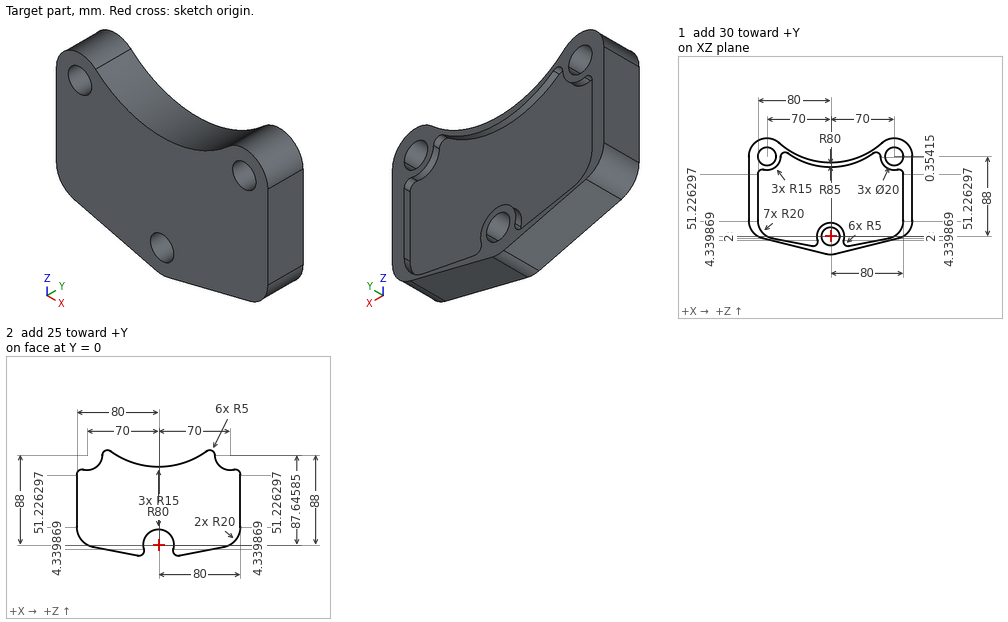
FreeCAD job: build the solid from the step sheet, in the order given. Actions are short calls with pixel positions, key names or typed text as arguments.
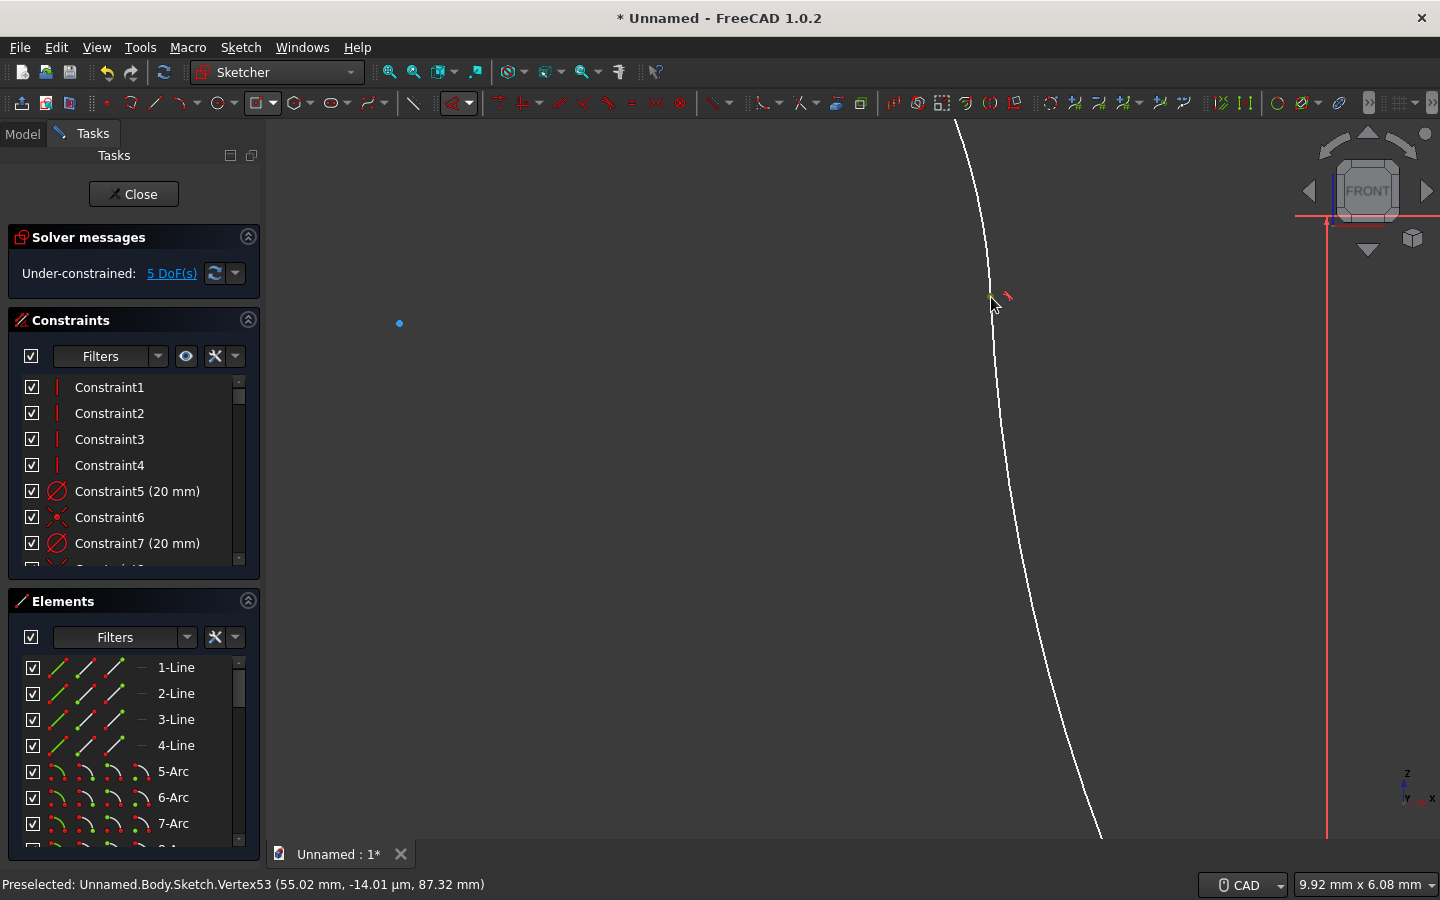
scroll(1053, 264, down, 16)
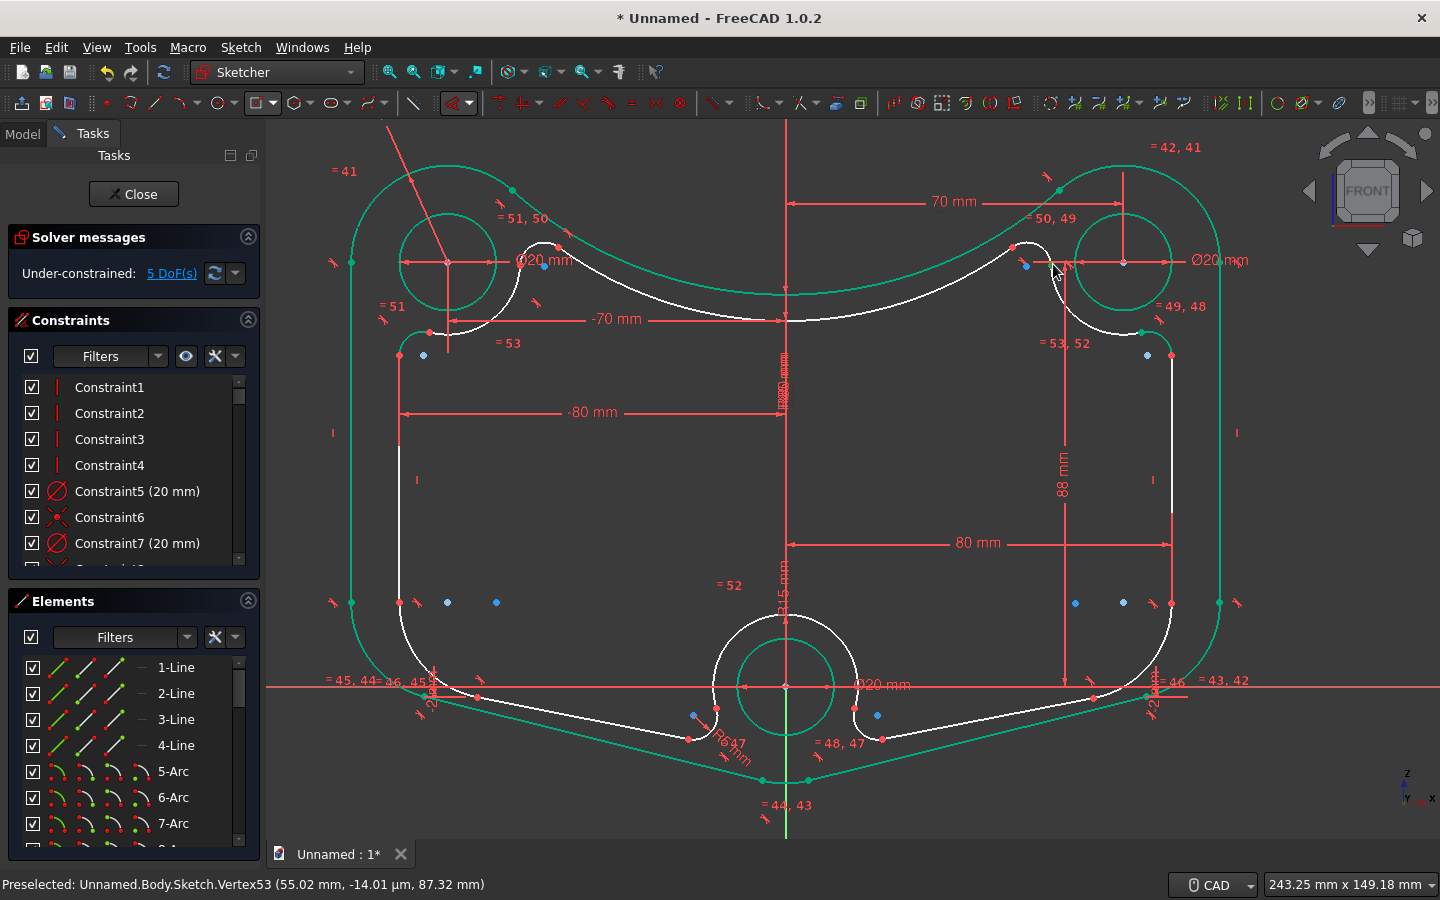
scroll(1123, 262, up, 16)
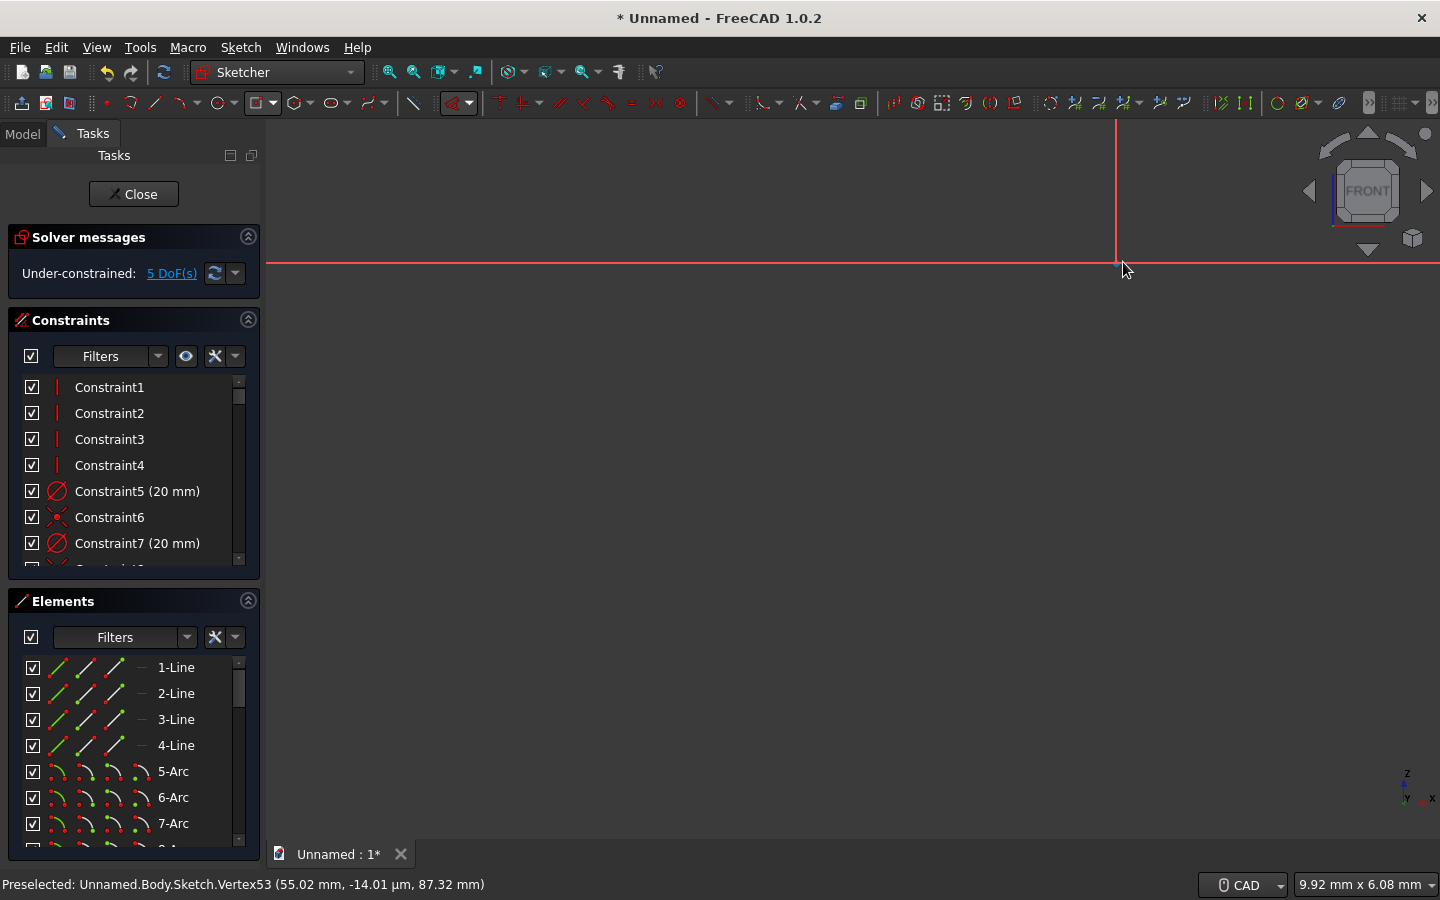
click(1116, 263)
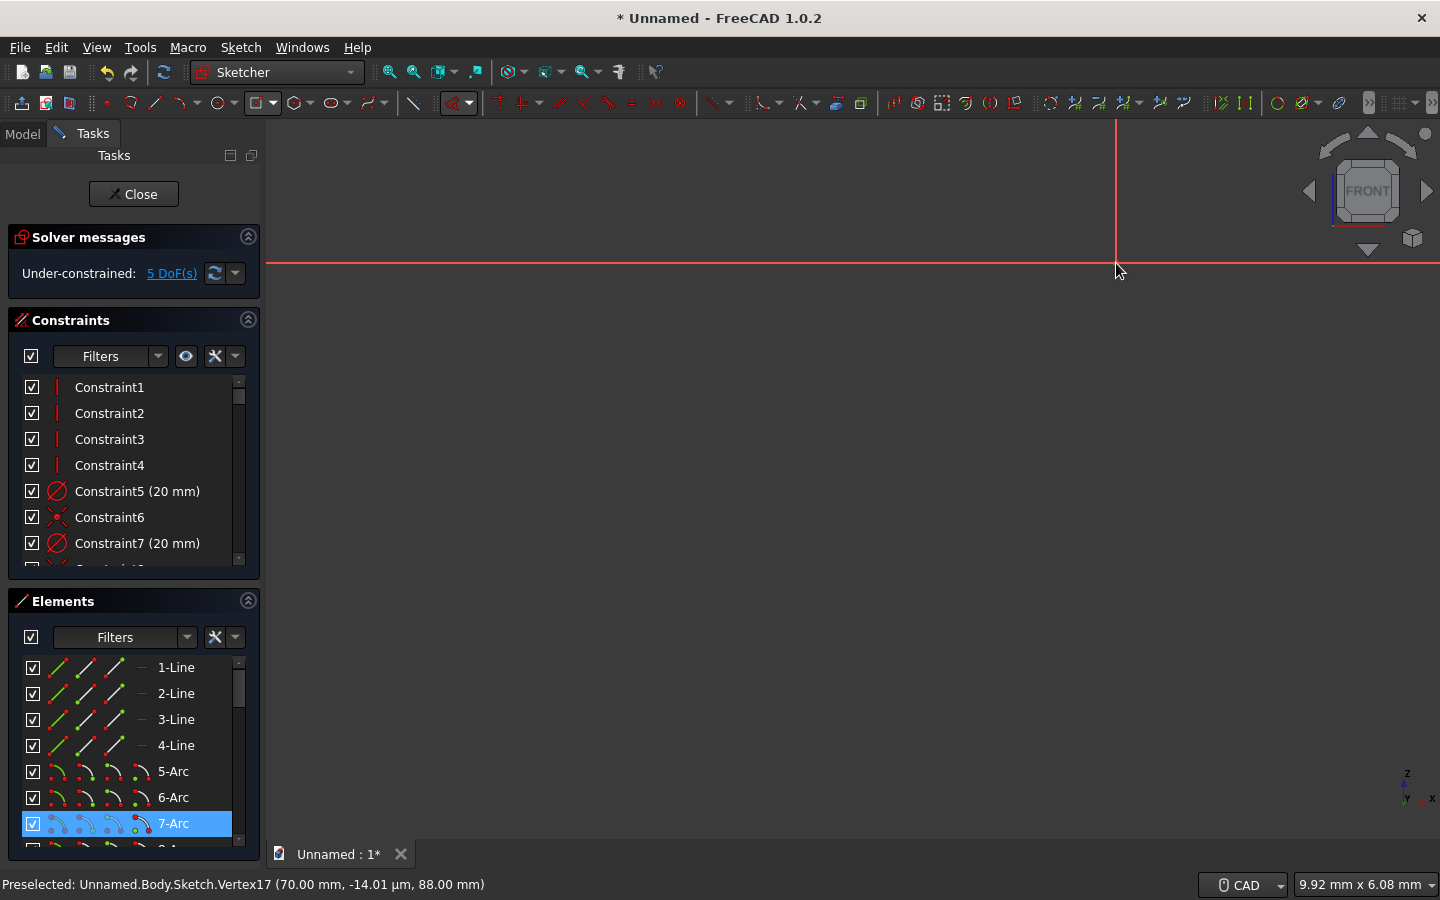
click(472, 104)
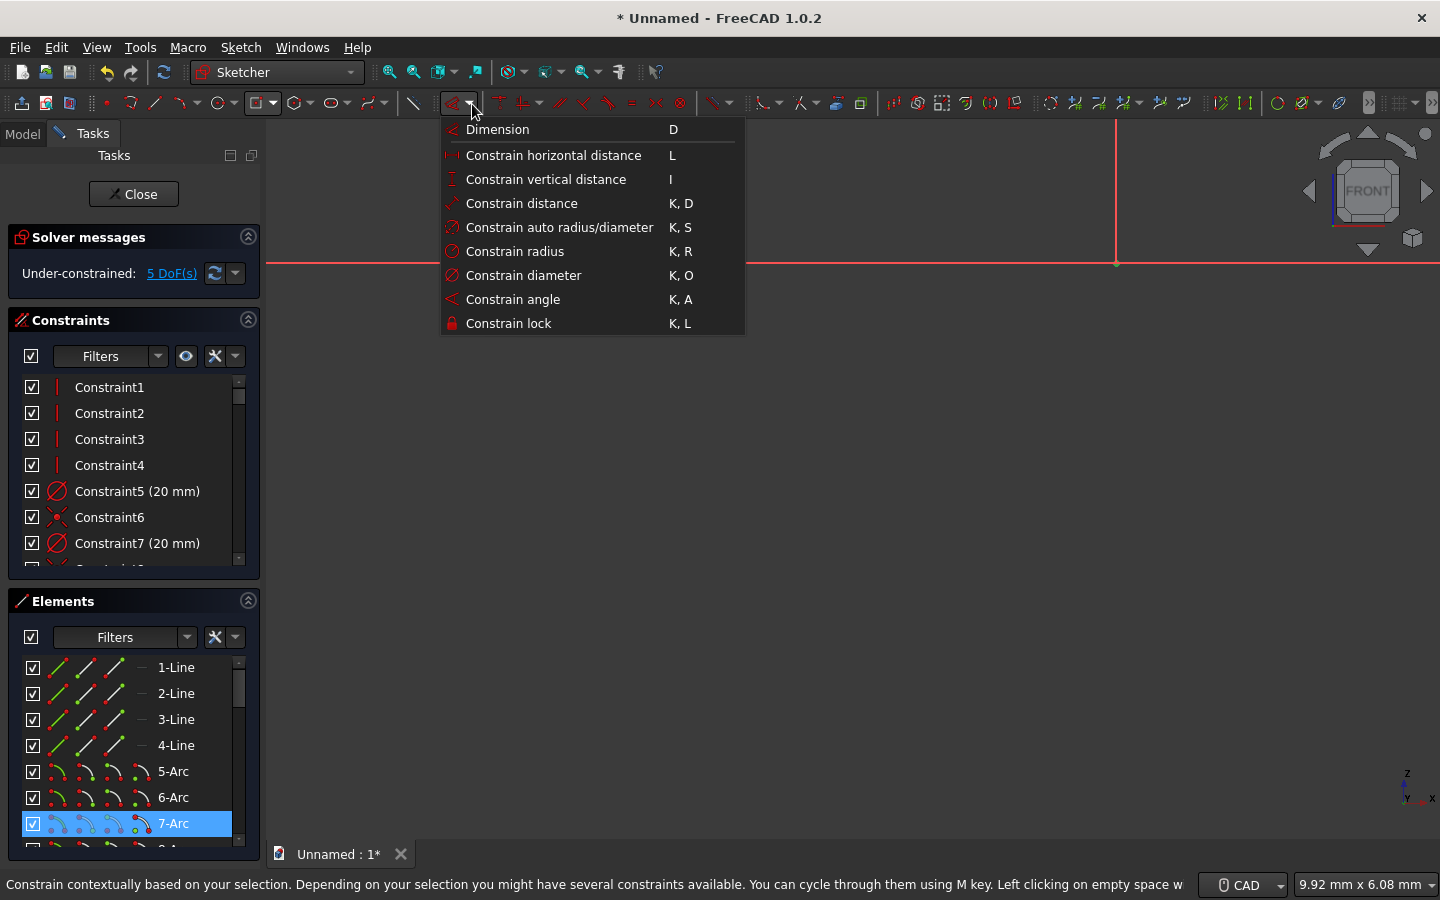
click(593, 179)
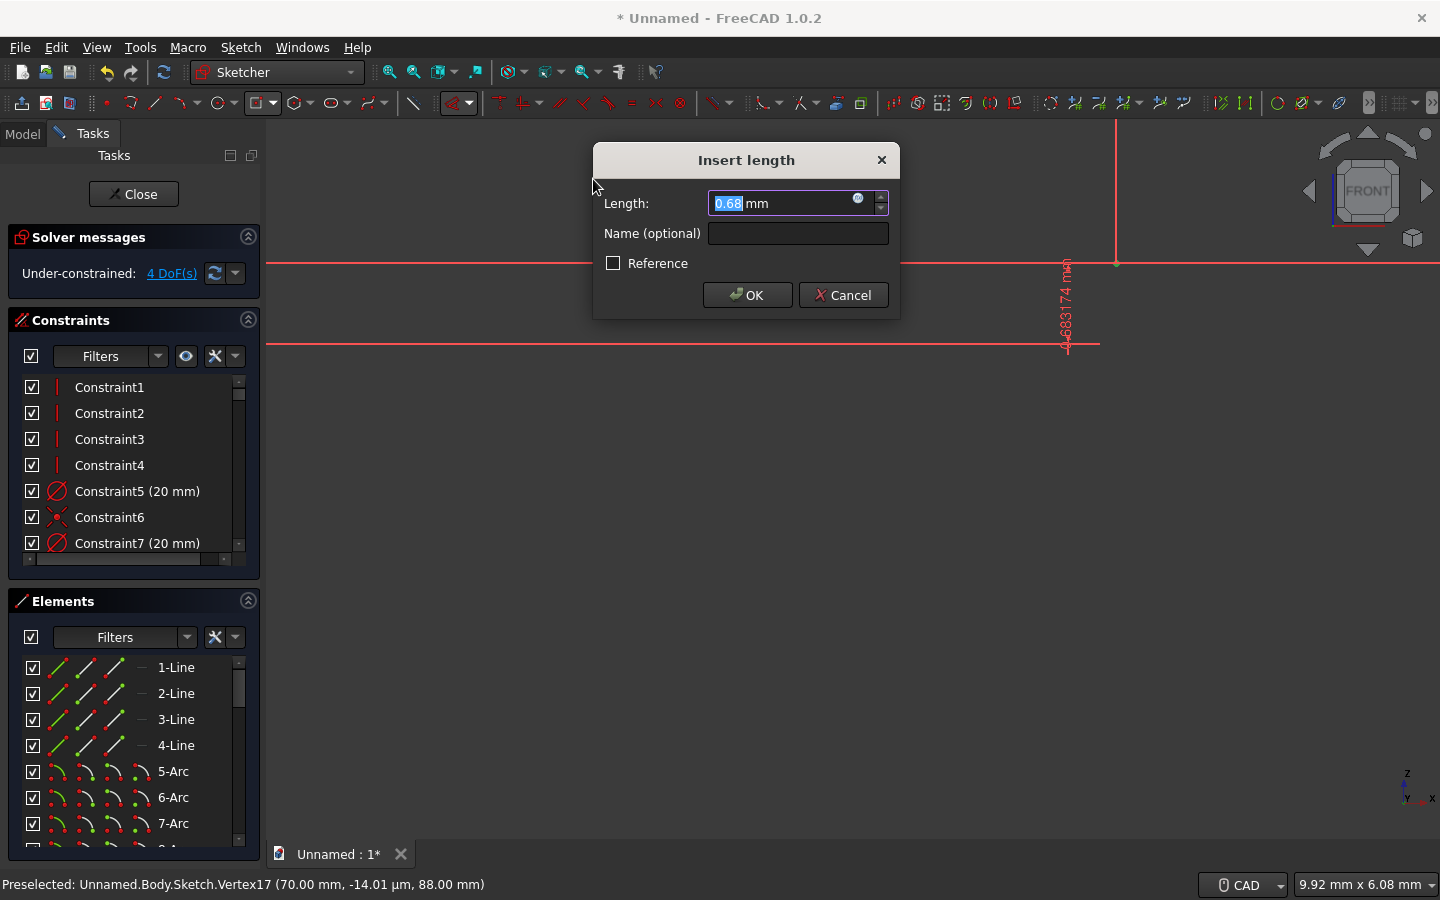
text(0.35415)
key(Return)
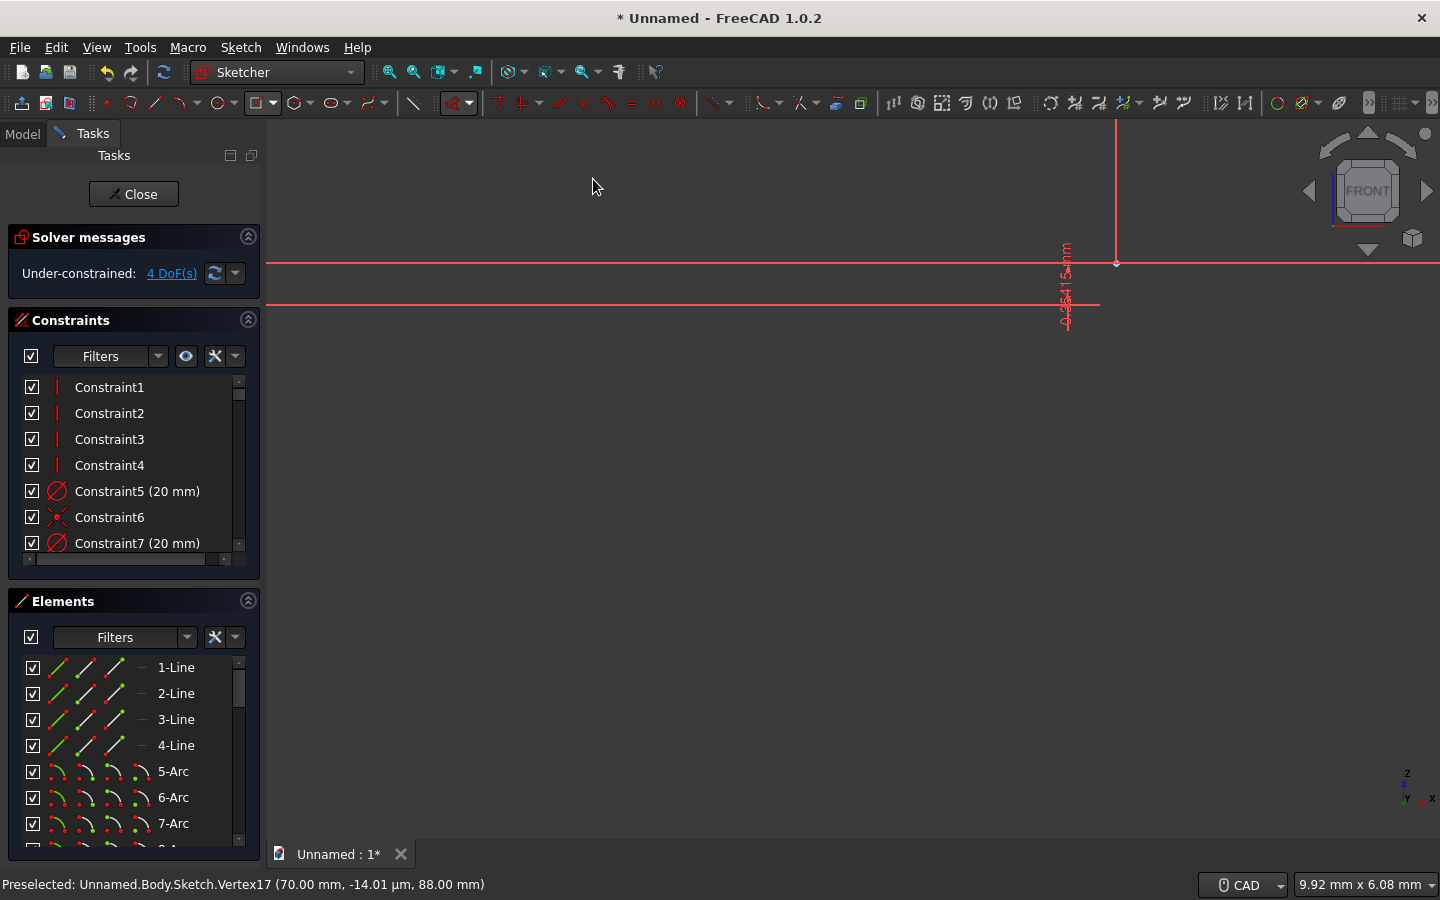
scroll(1123, 262, down, 16)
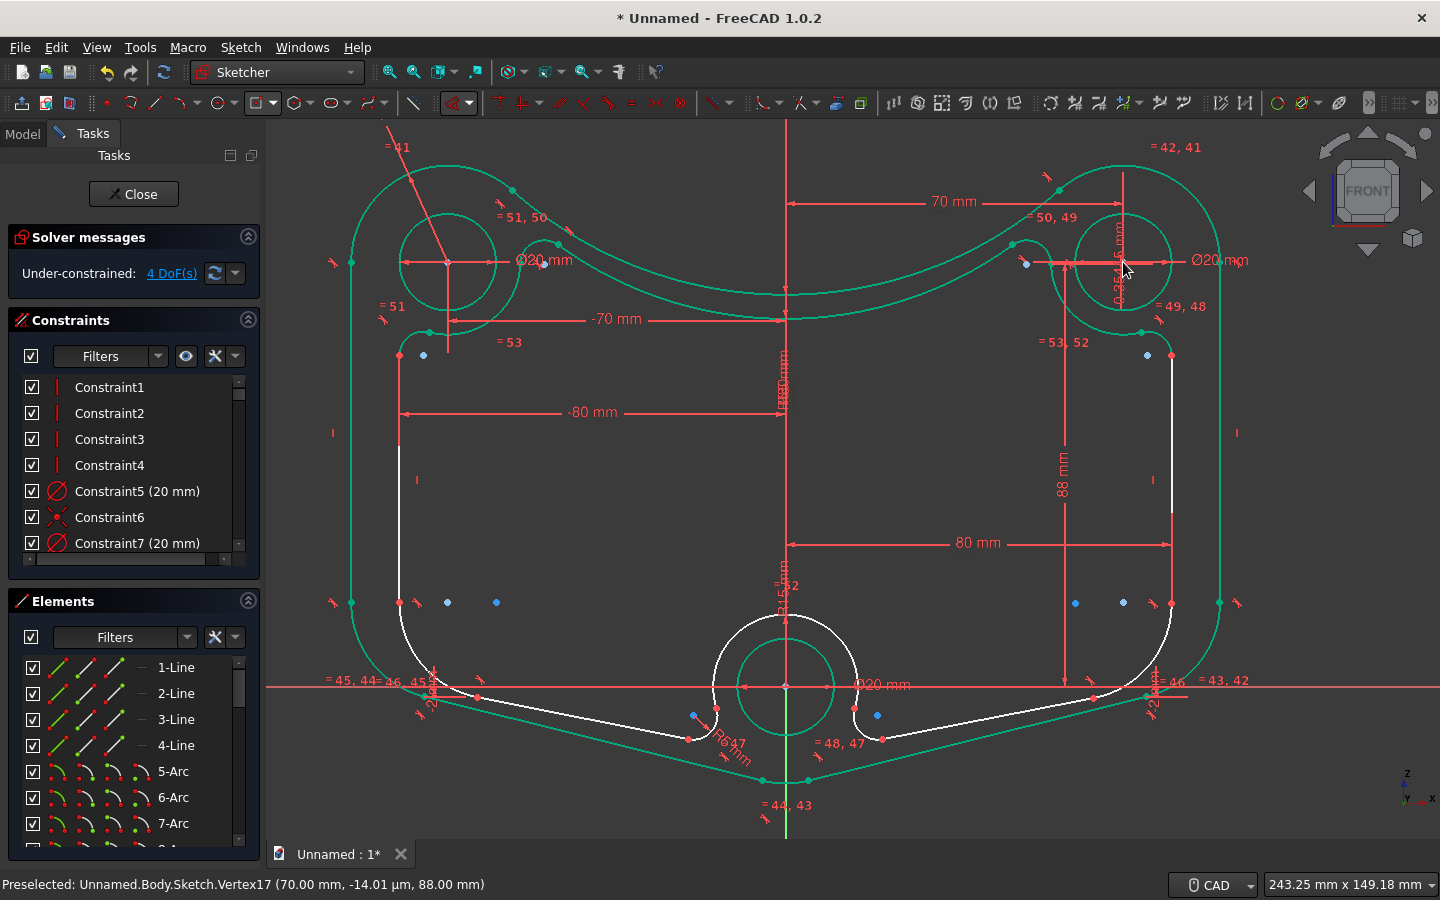
click(399, 430)